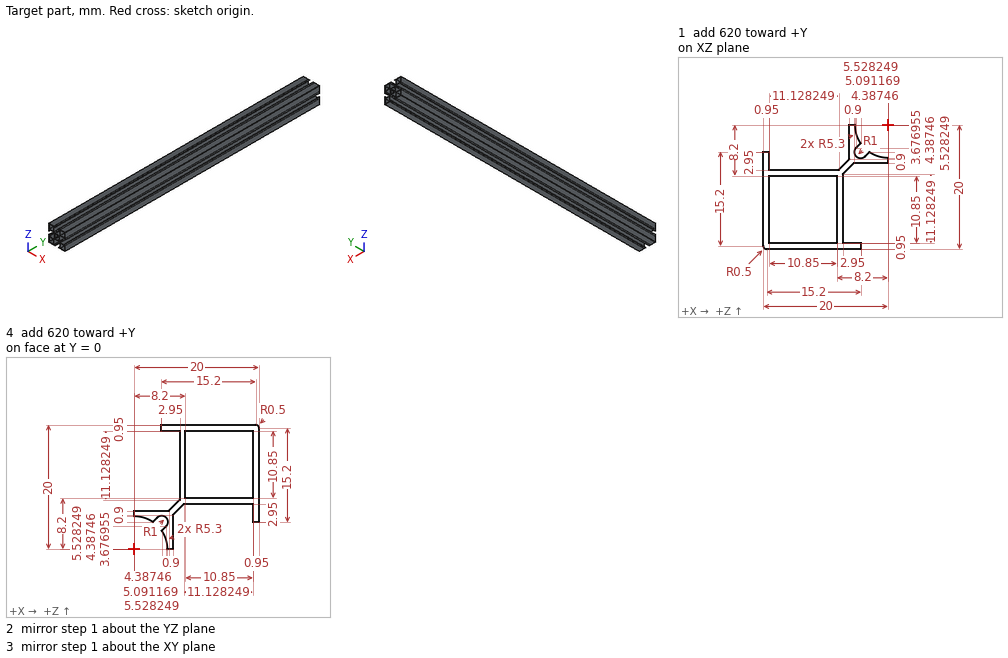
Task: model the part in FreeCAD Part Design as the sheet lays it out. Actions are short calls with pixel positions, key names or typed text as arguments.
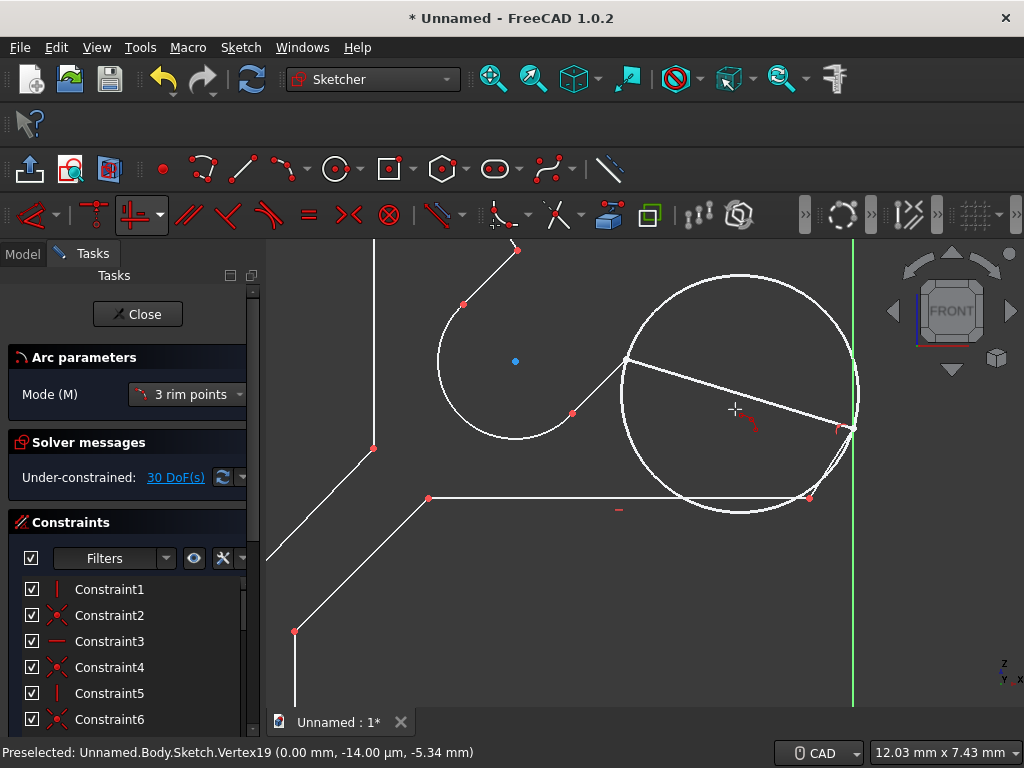
click(734, 408)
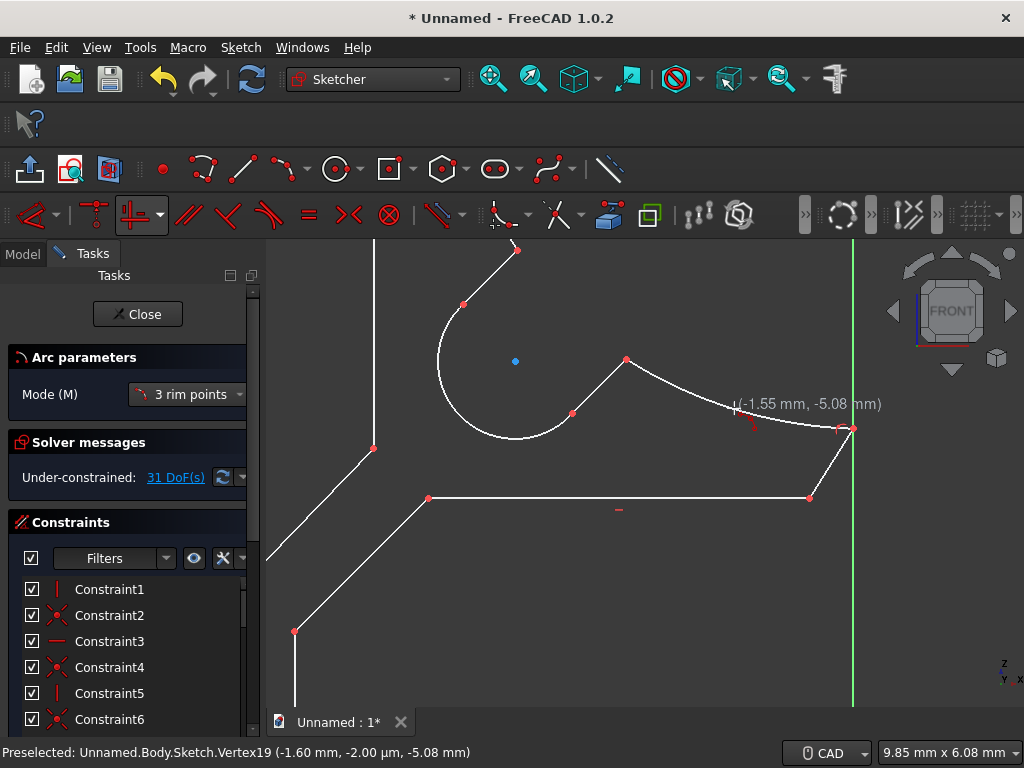
scroll(701, 393, down, 8)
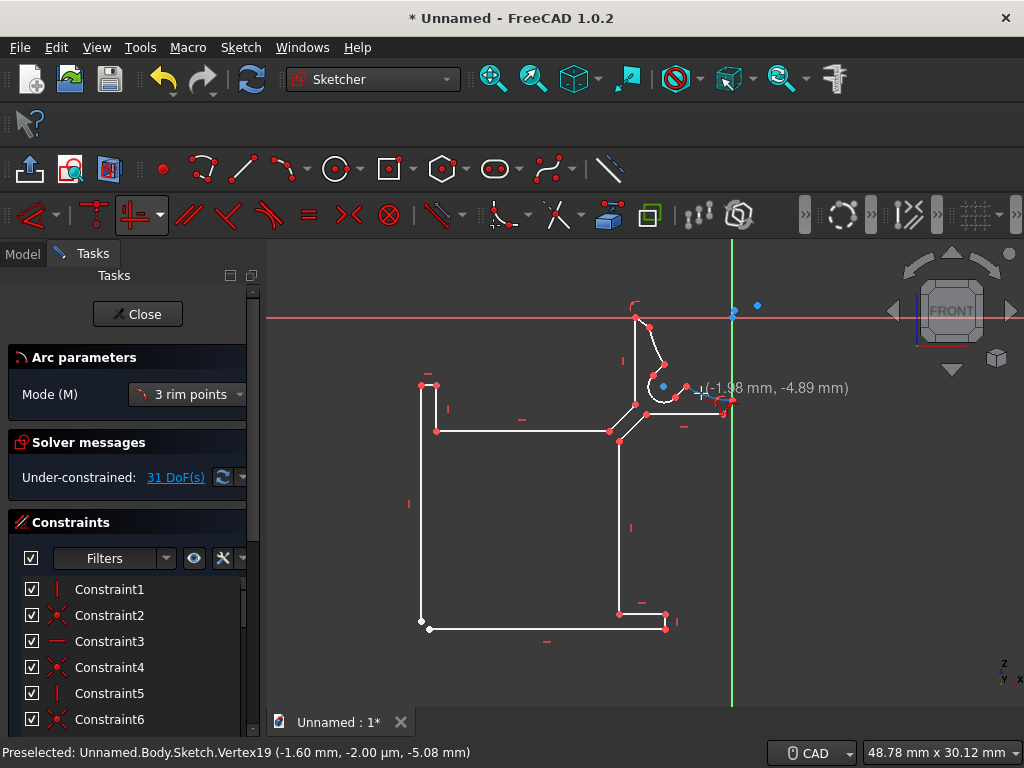
scroll(429, 628, up, 2)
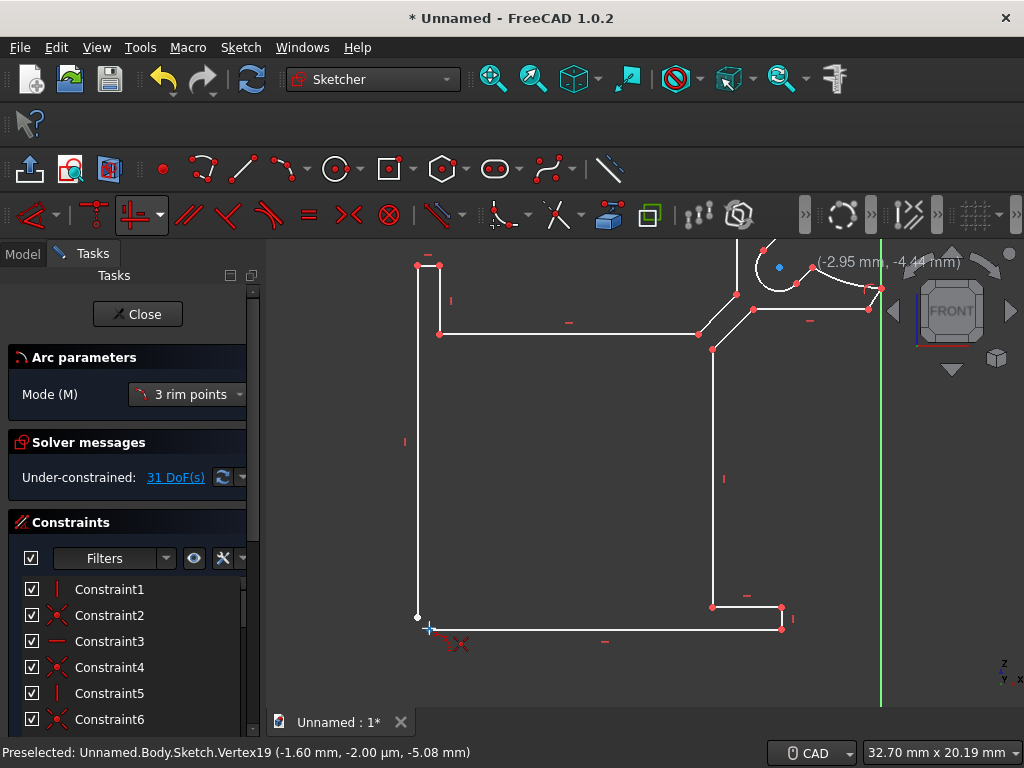
click(430, 630)
click(418, 618)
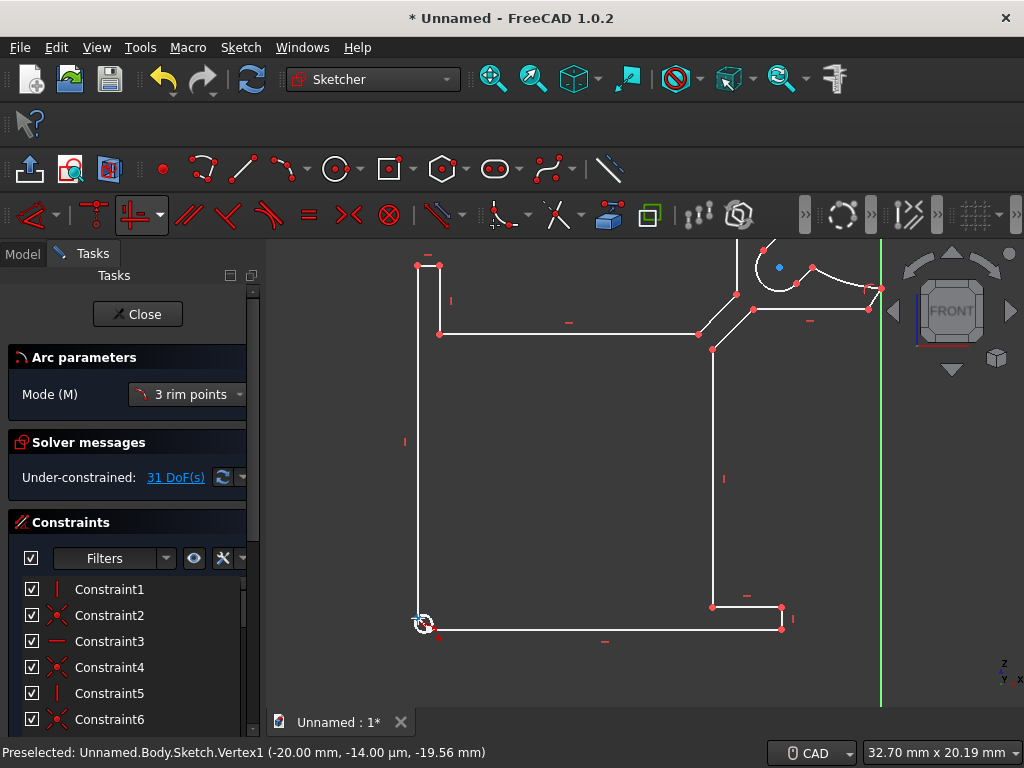
scroll(421, 625, up, 8)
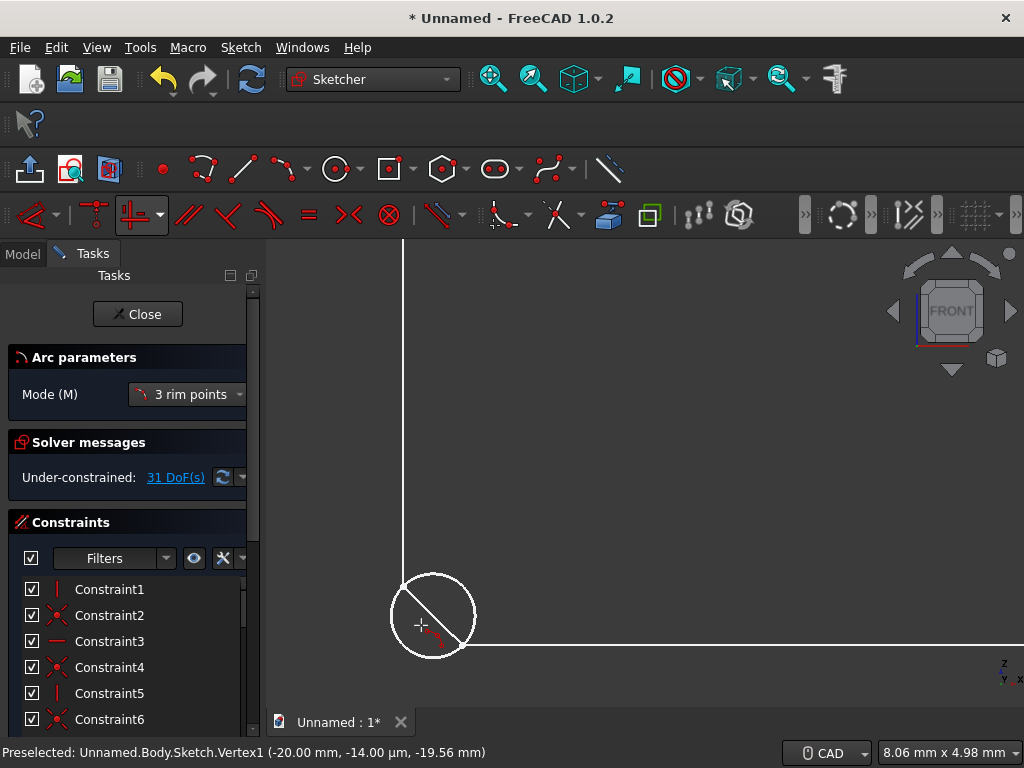
click(420, 620)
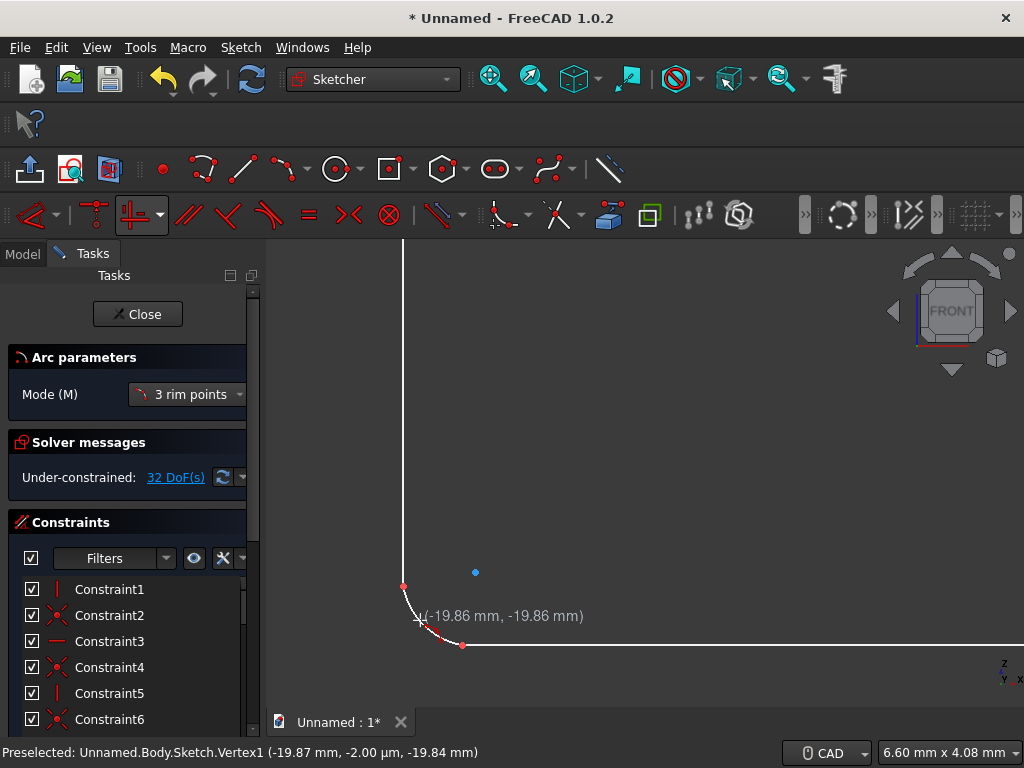
key(g)
key(r)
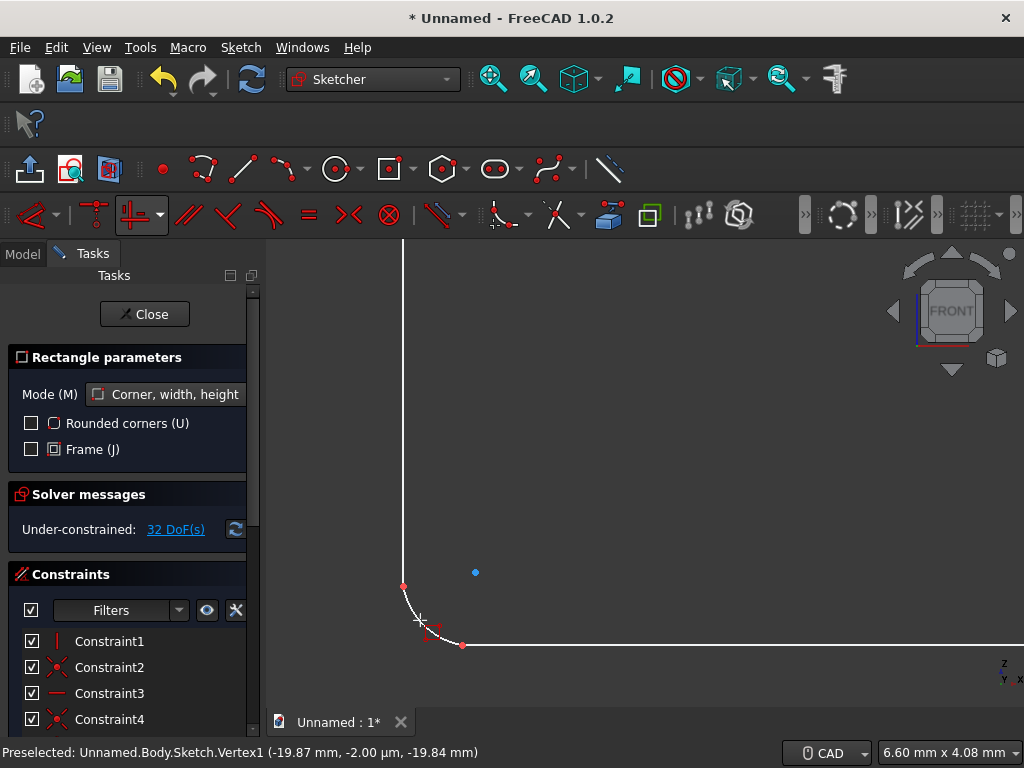
scroll(424, 627, down, 10)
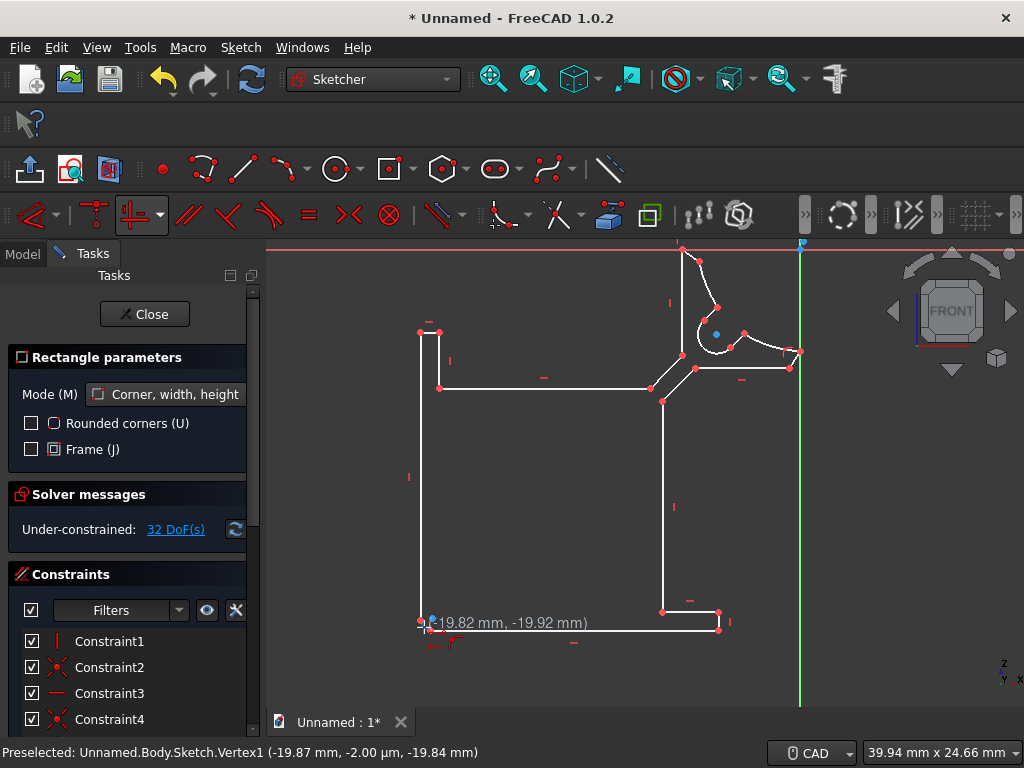
click(436, 446)
move(605, 614)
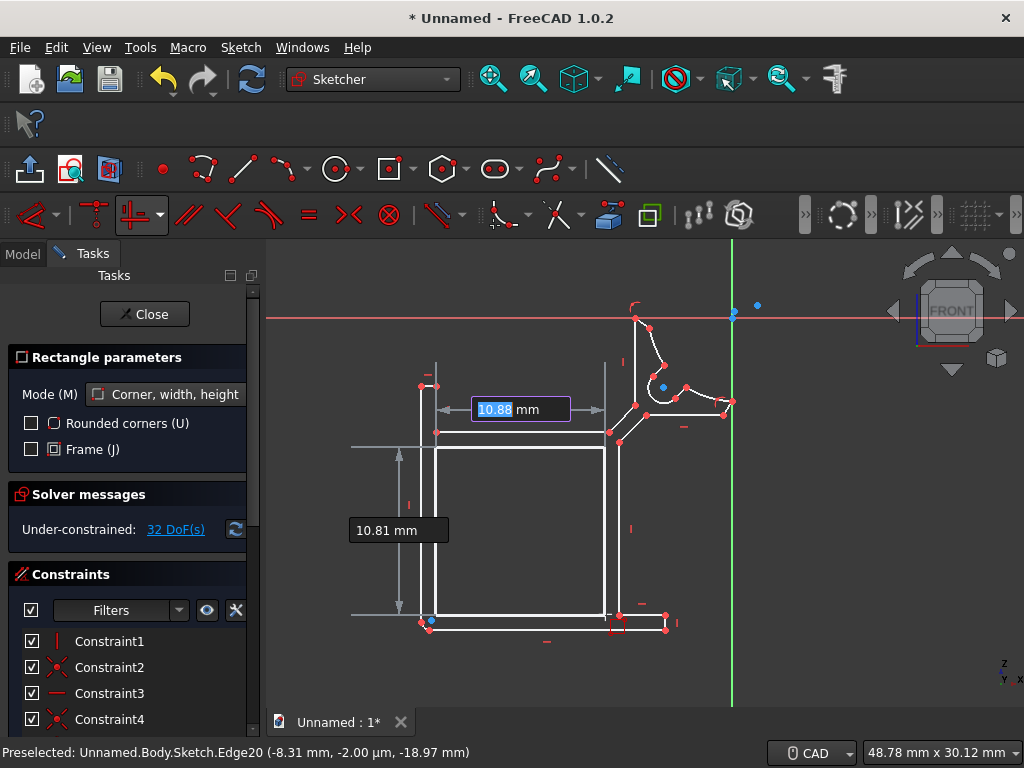
text(10.85)
key(Tab)
text(10.85)
key(Return)
key(Escape)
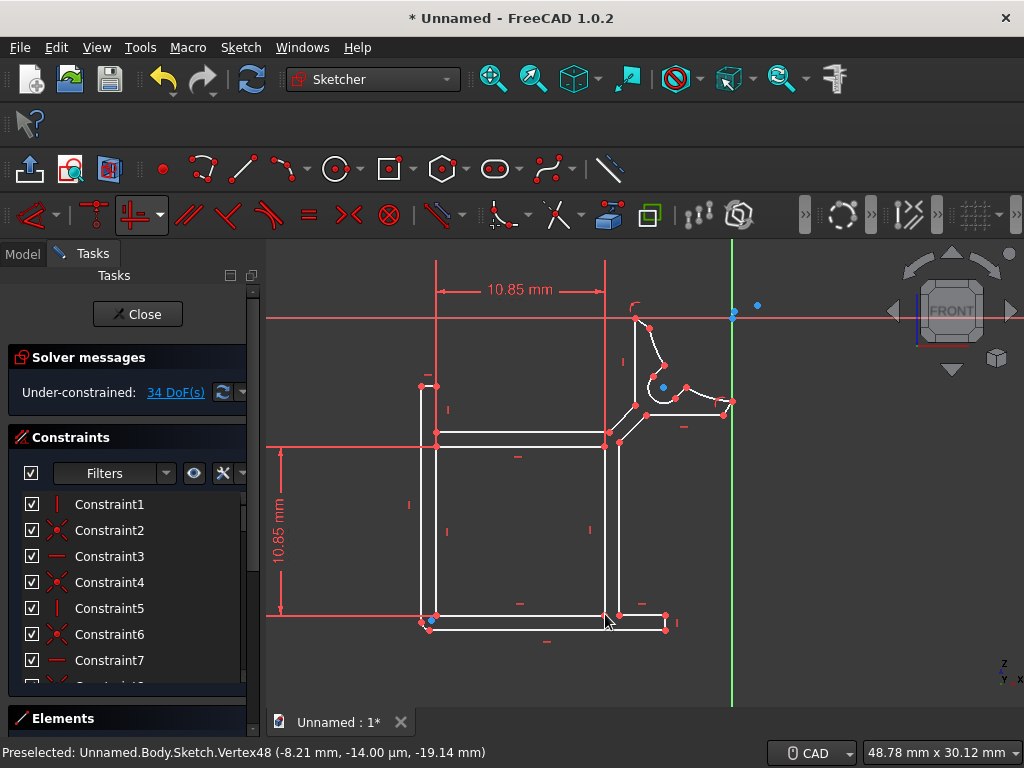
click(421, 551)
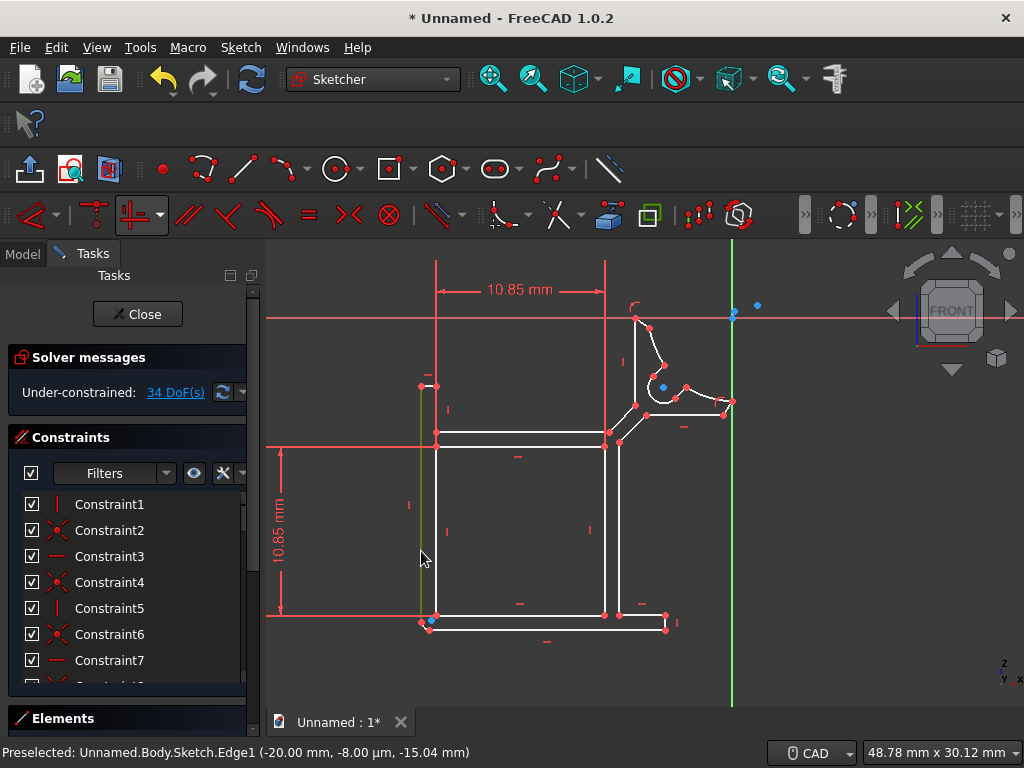
scroll(424, 627, up, 5)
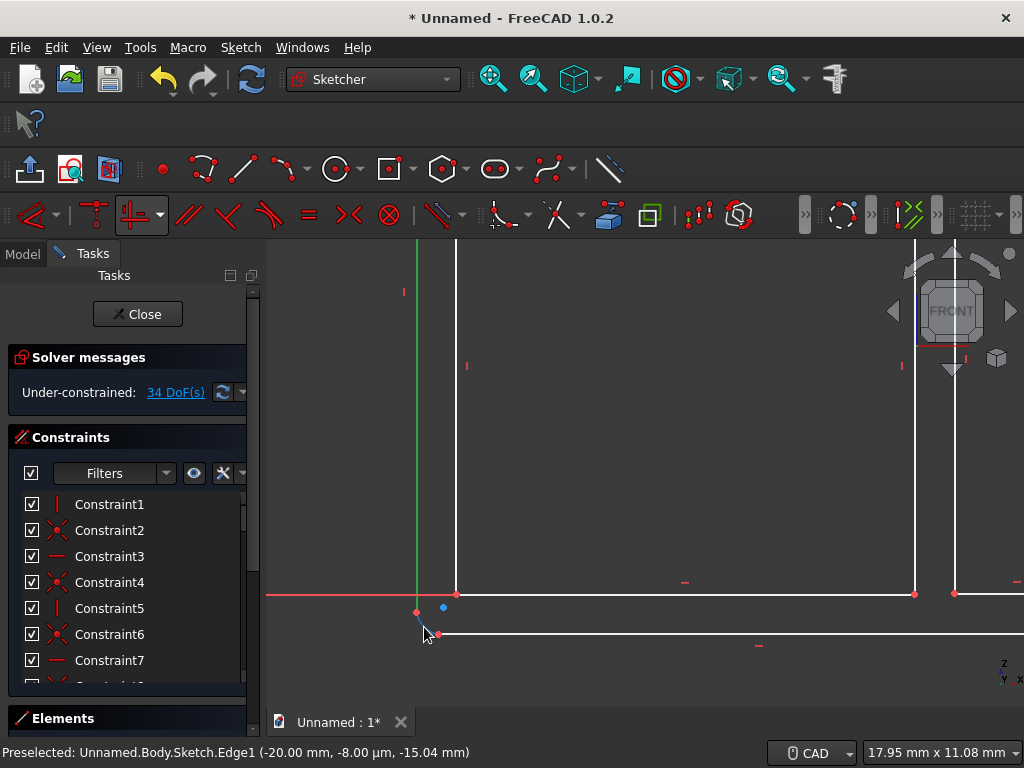
click(424, 627)